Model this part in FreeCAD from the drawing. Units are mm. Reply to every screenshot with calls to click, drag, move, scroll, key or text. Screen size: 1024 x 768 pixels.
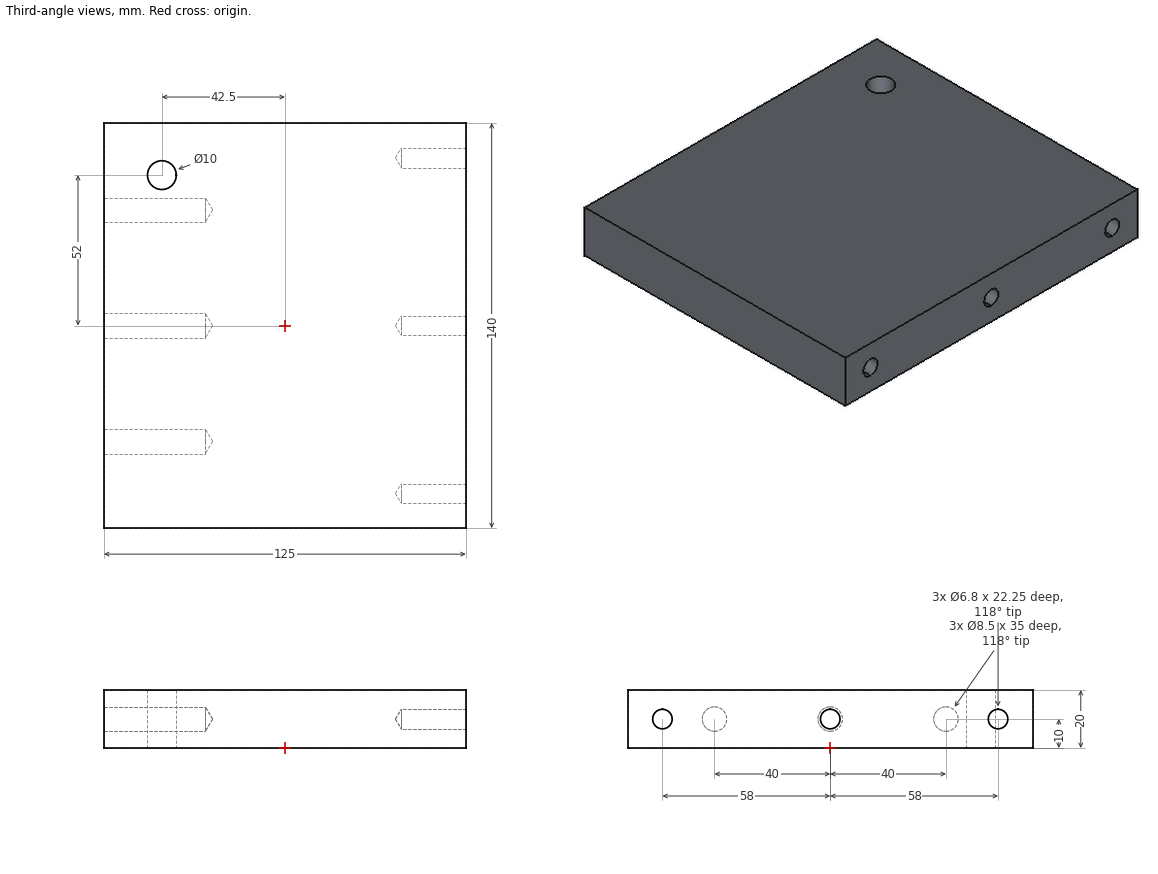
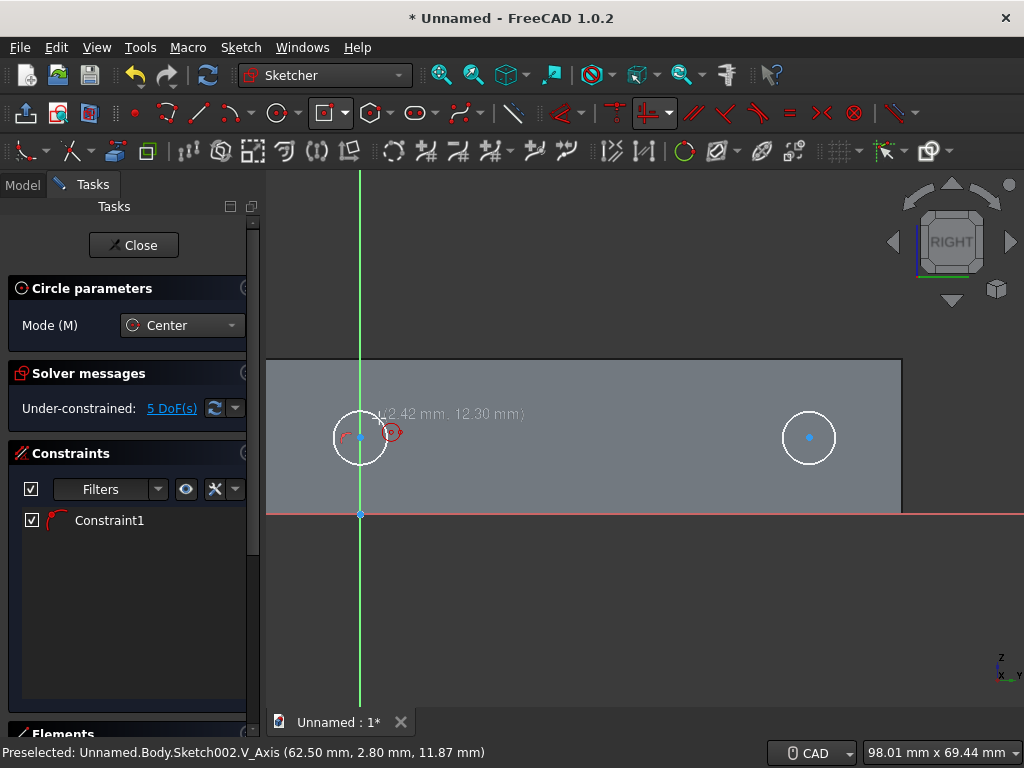
scroll(753, 419, down, 4)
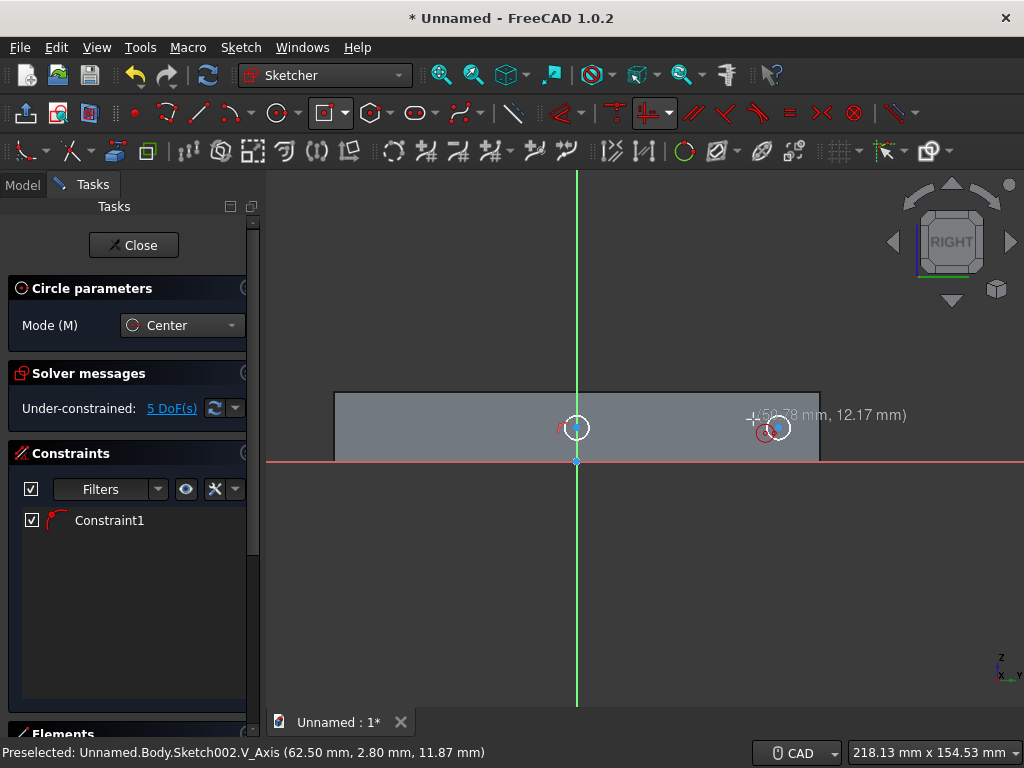
scroll(375, 427, up, 4)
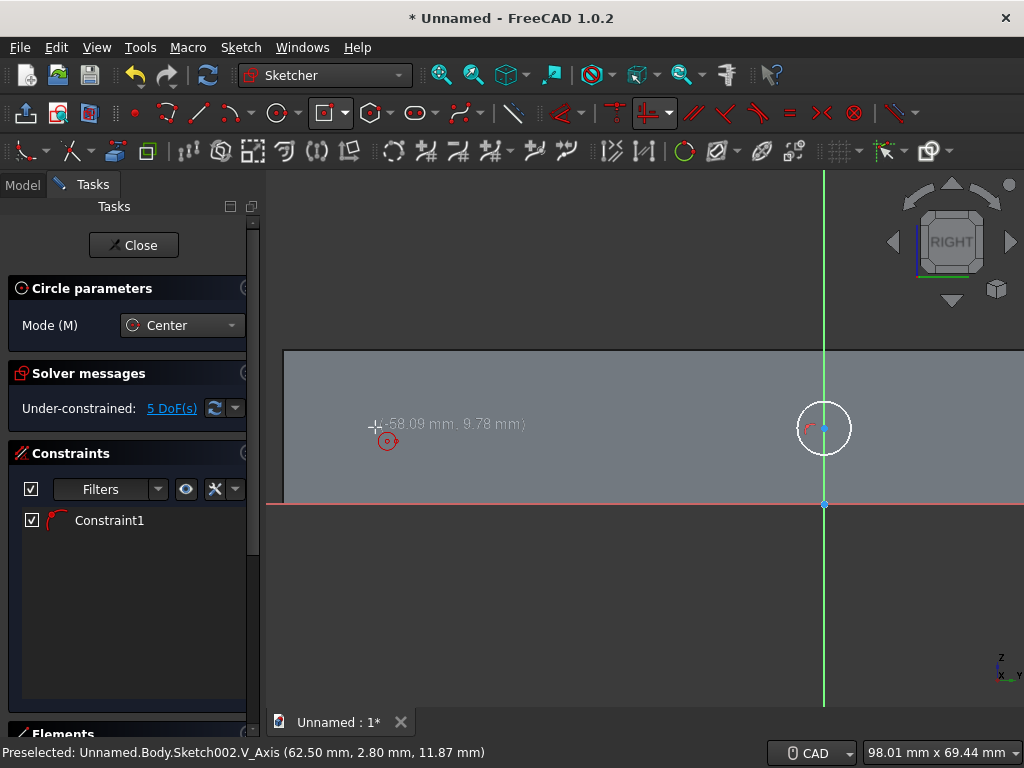
click(376, 427)
click(394, 408)
key(Escape)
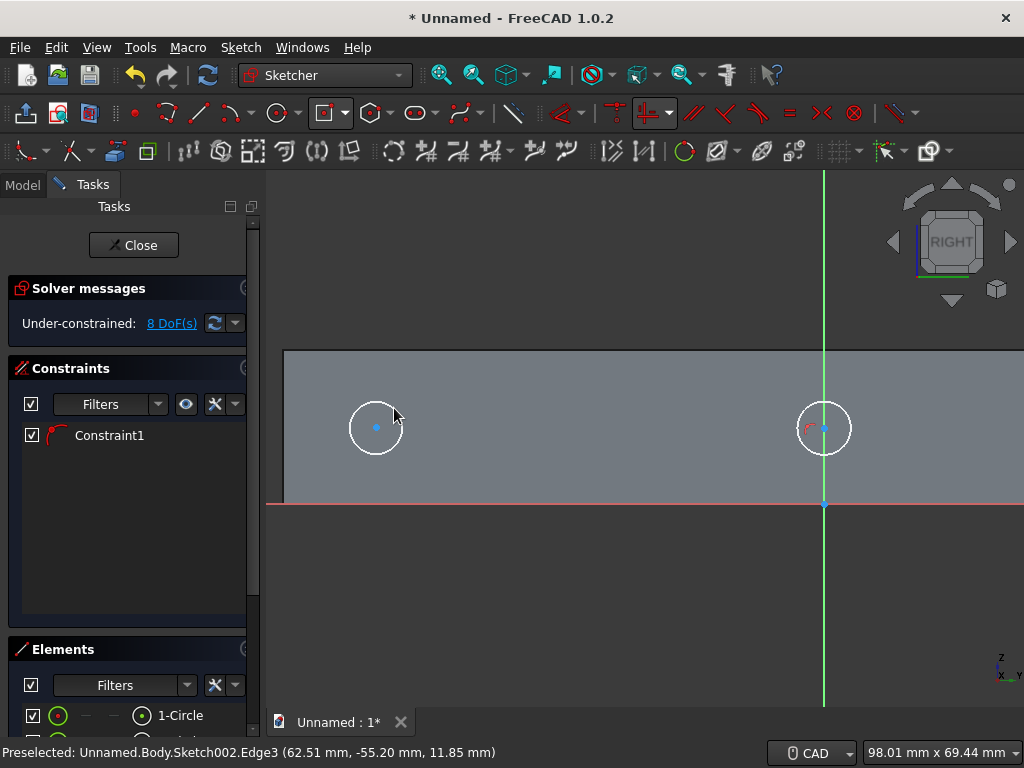
scroll(374, 427, down, 4)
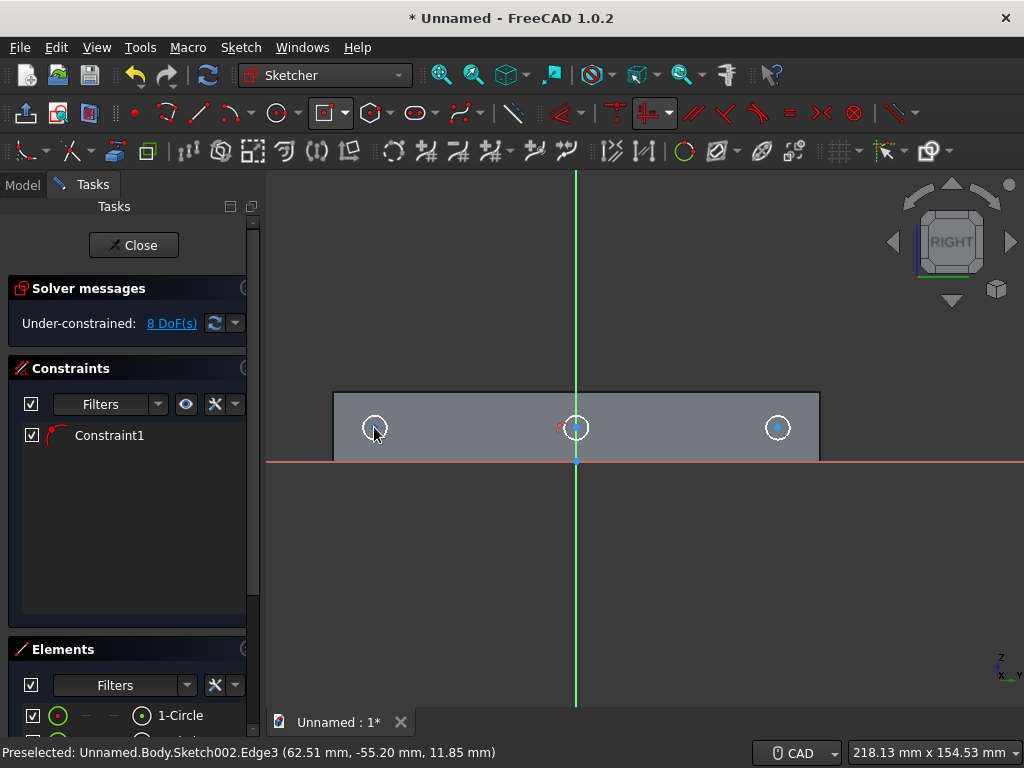
click(786, 419)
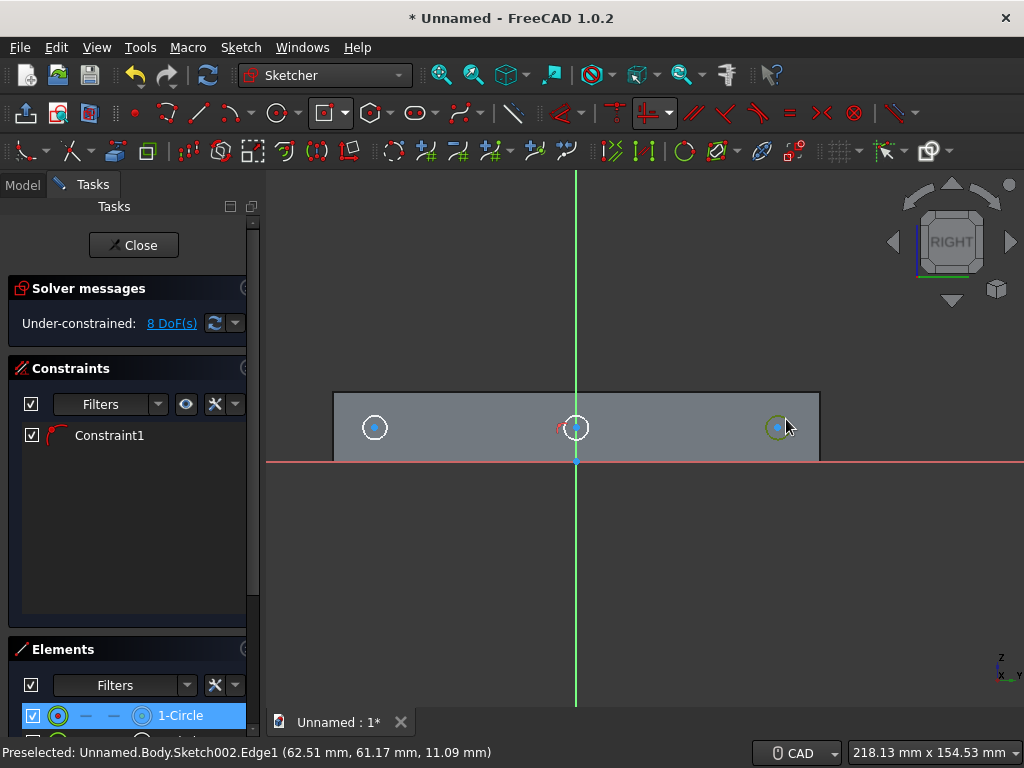
click(577, 416)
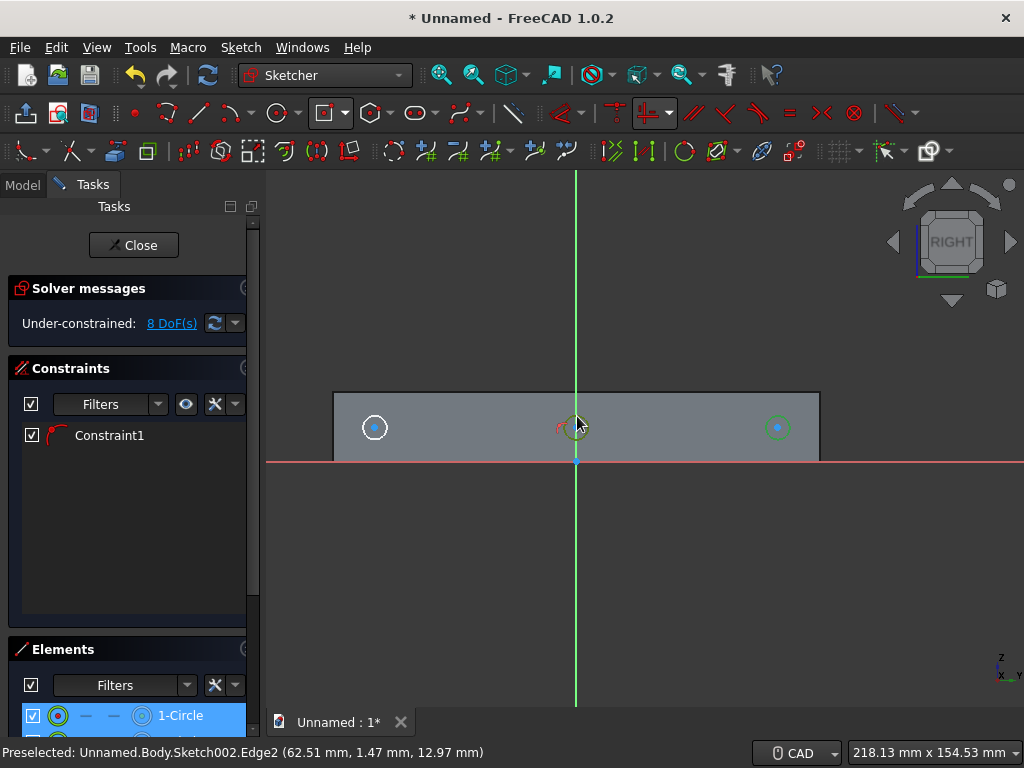
click(383, 419)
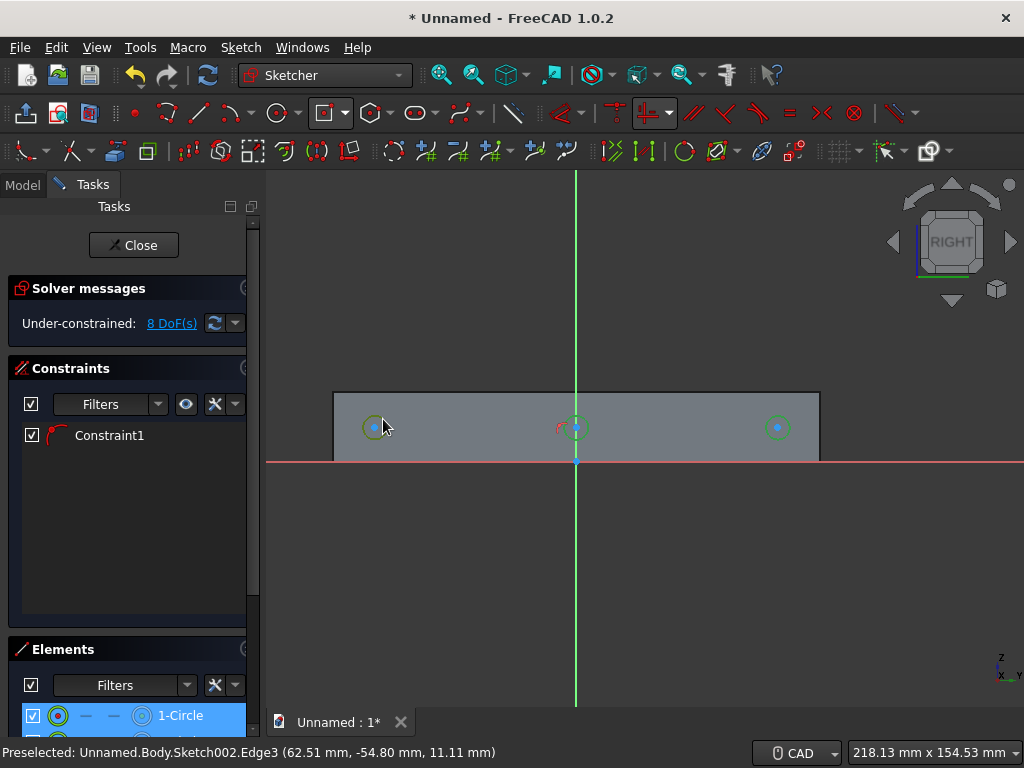
click(790, 114)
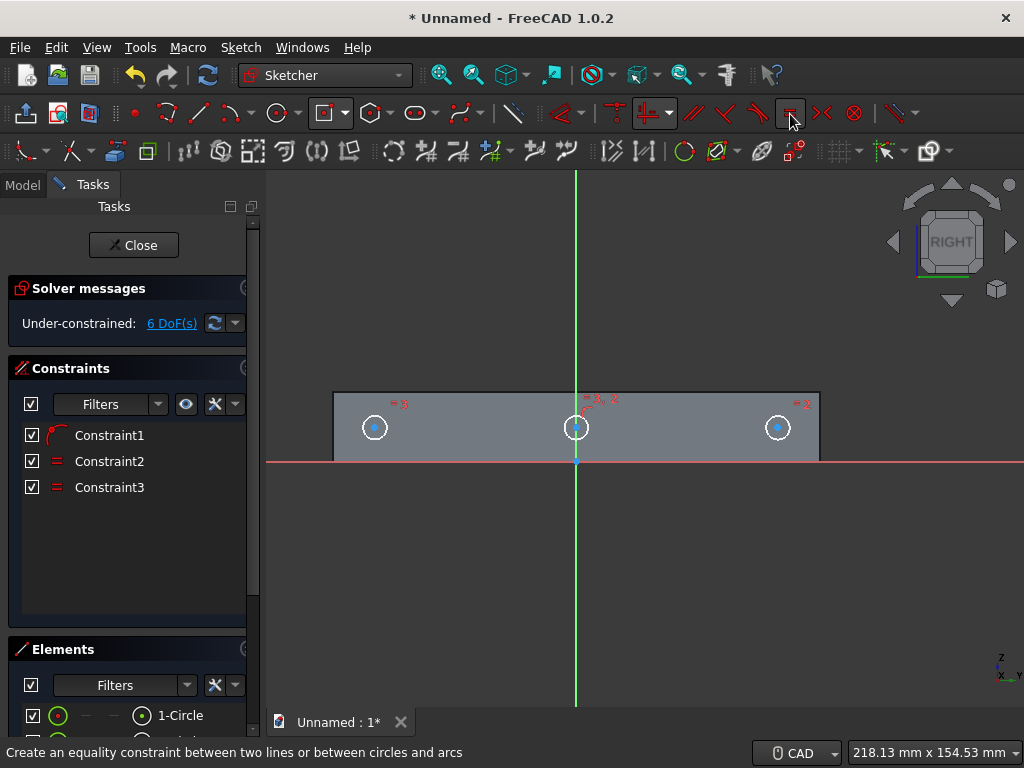
click(778, 428)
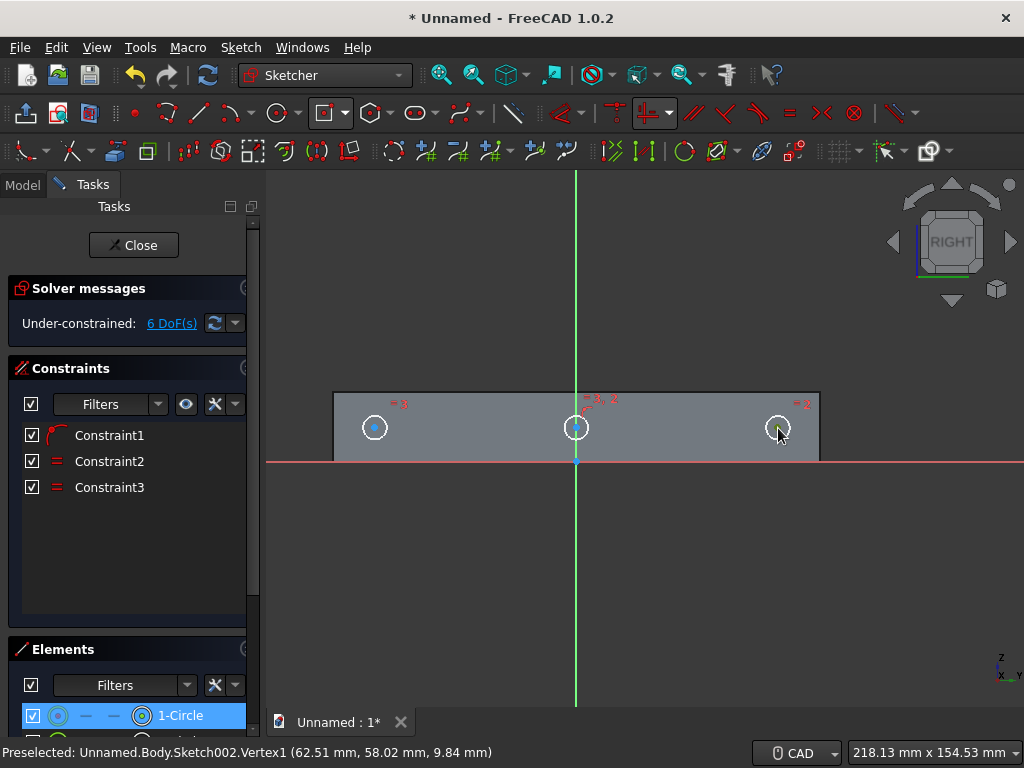
click(576, 428)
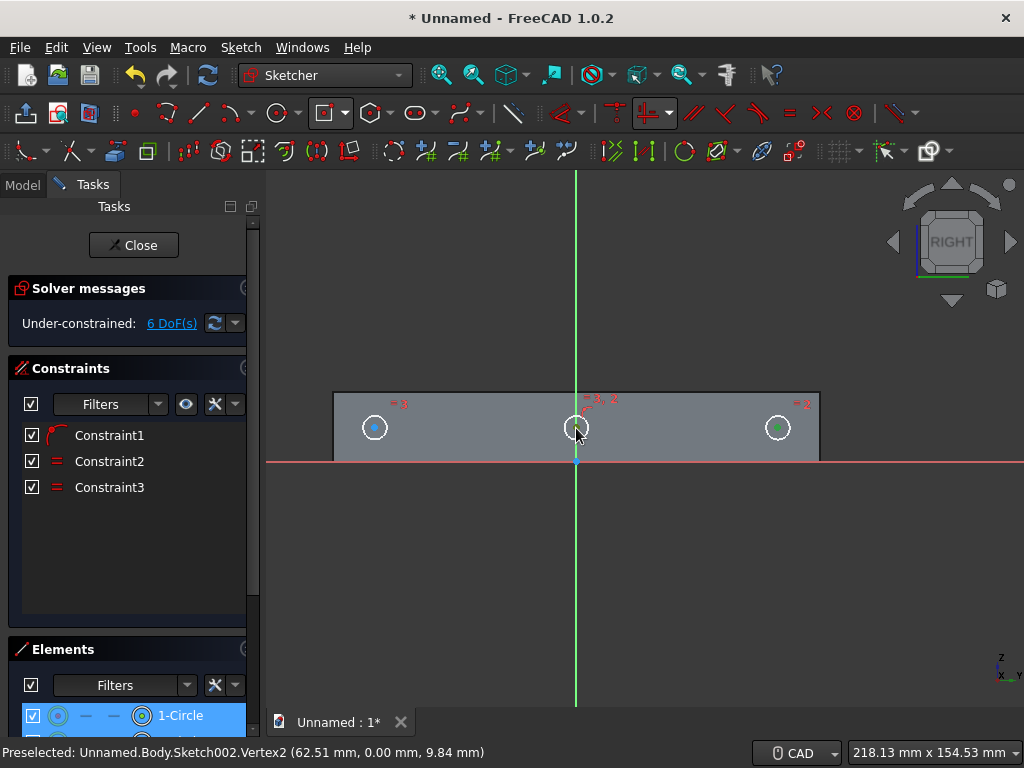
key(h)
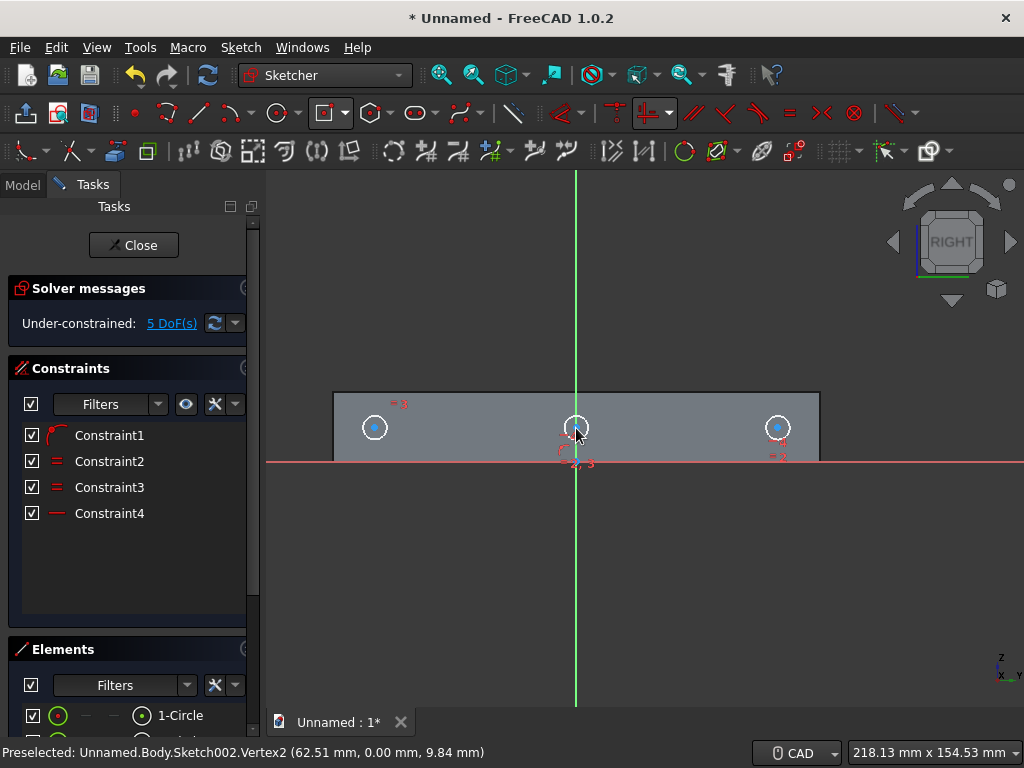
click(574, 426)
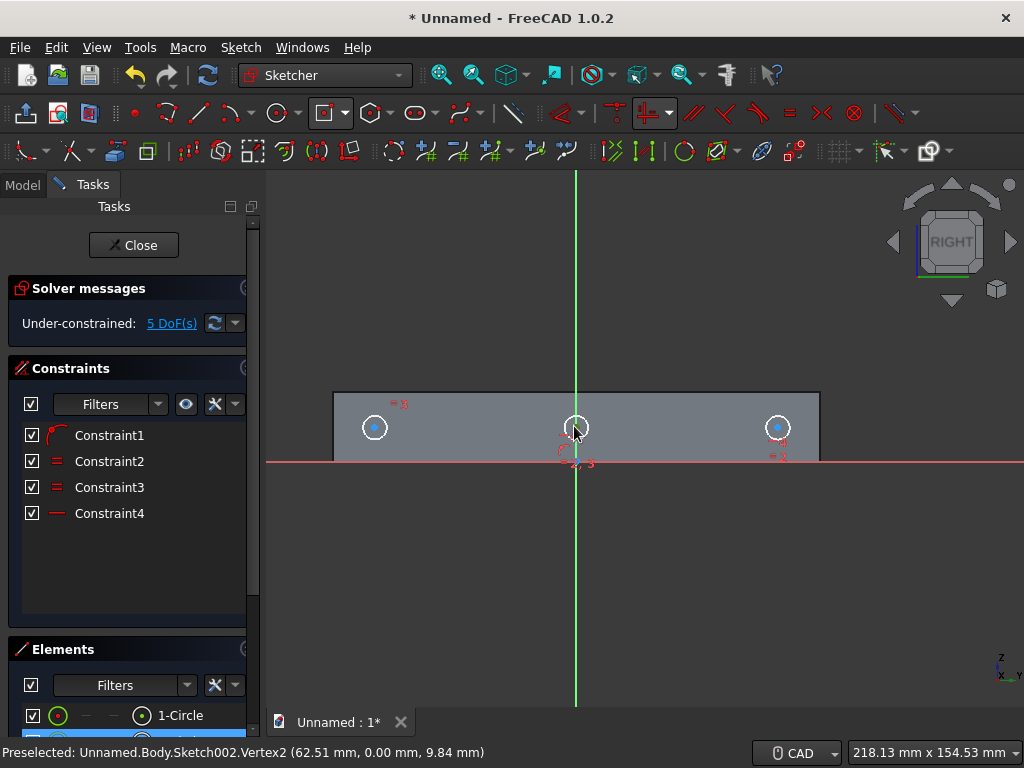
click(375, 428)